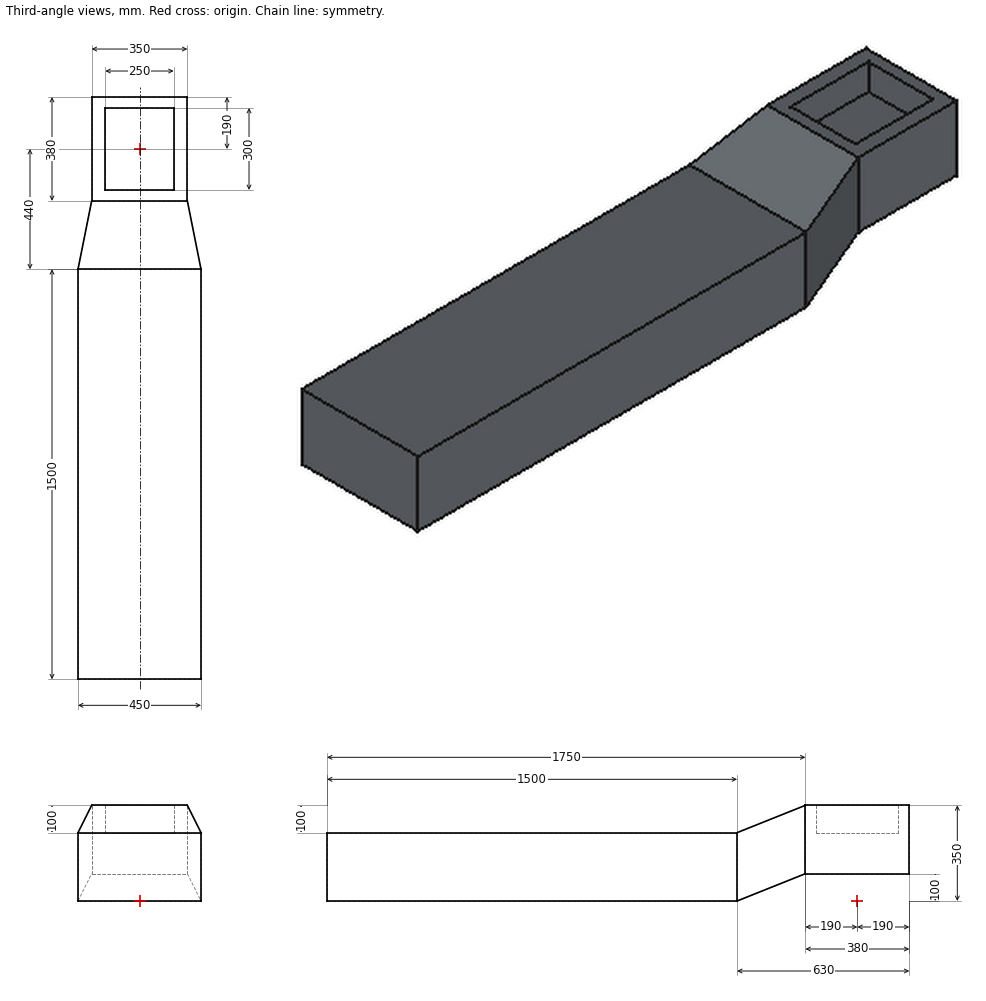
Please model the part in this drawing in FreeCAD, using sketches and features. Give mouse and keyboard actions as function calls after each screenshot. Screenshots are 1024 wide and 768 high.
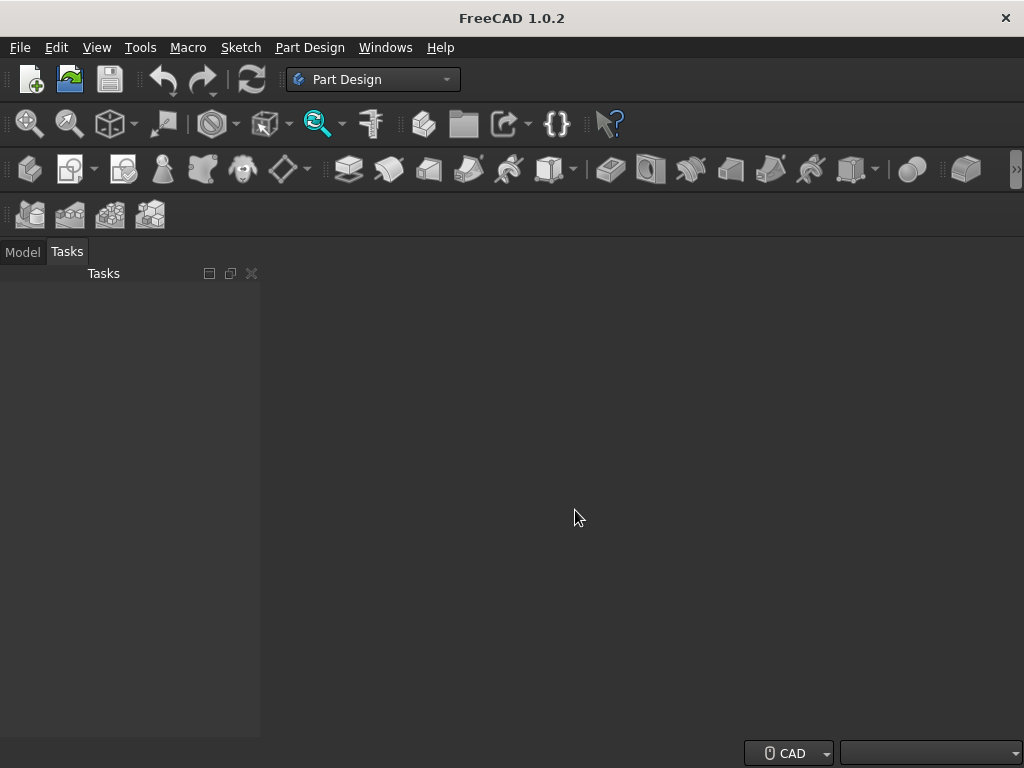
click(30, 80)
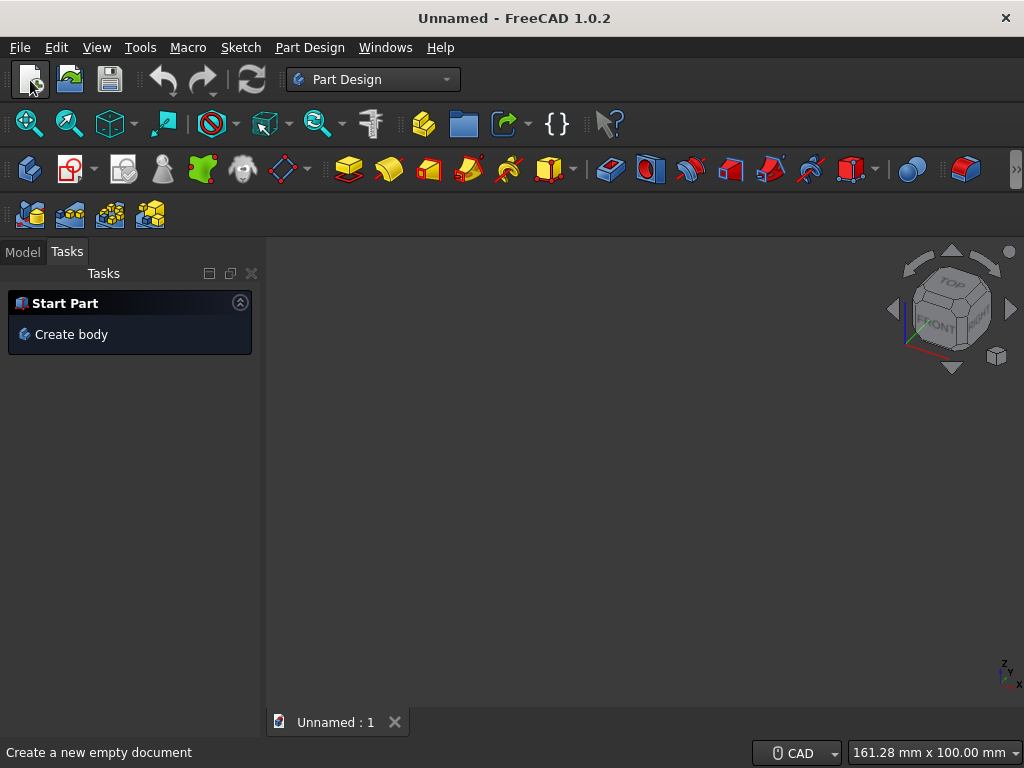
click(70, 170)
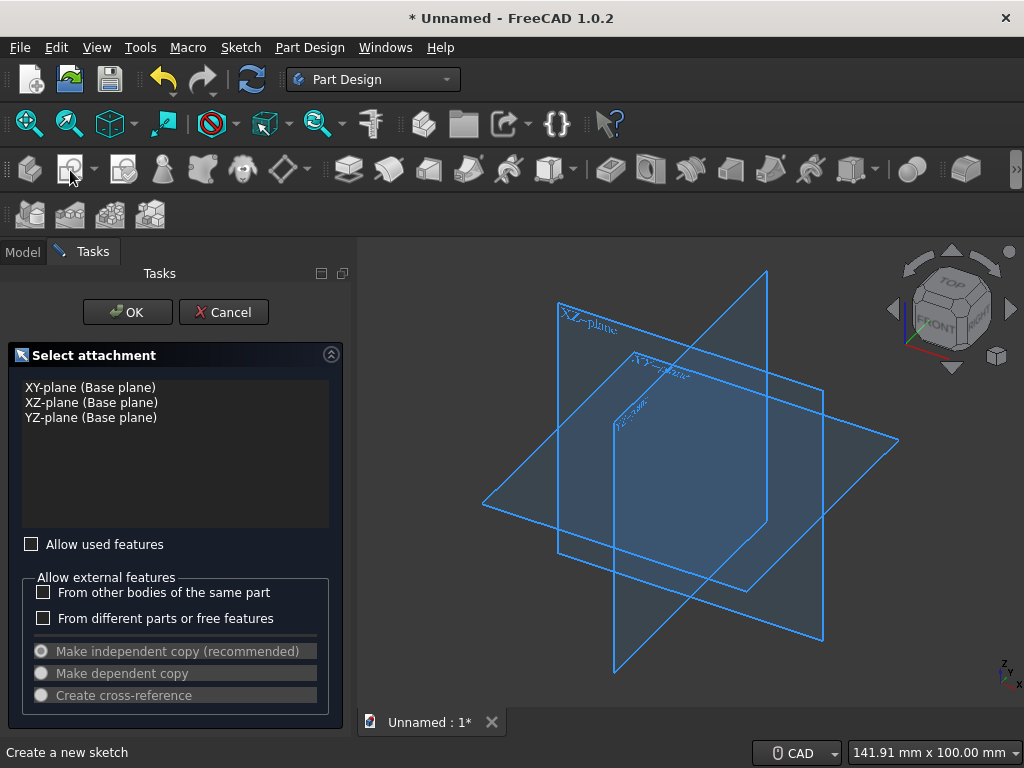
click(82, 388)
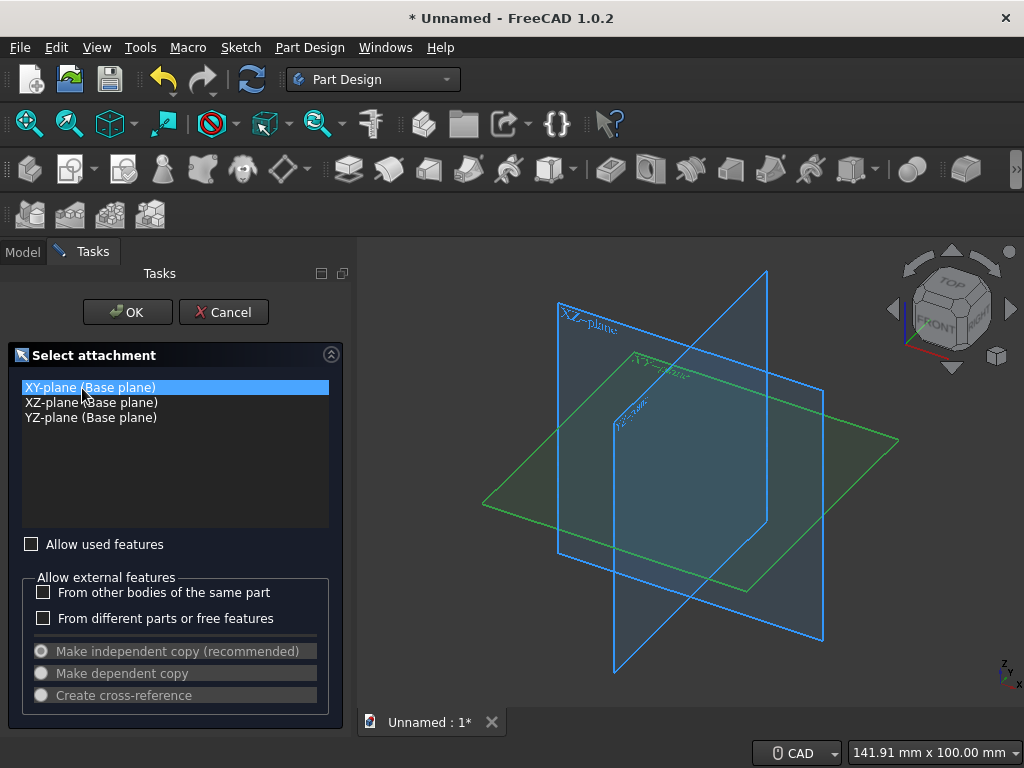
click(128, 312)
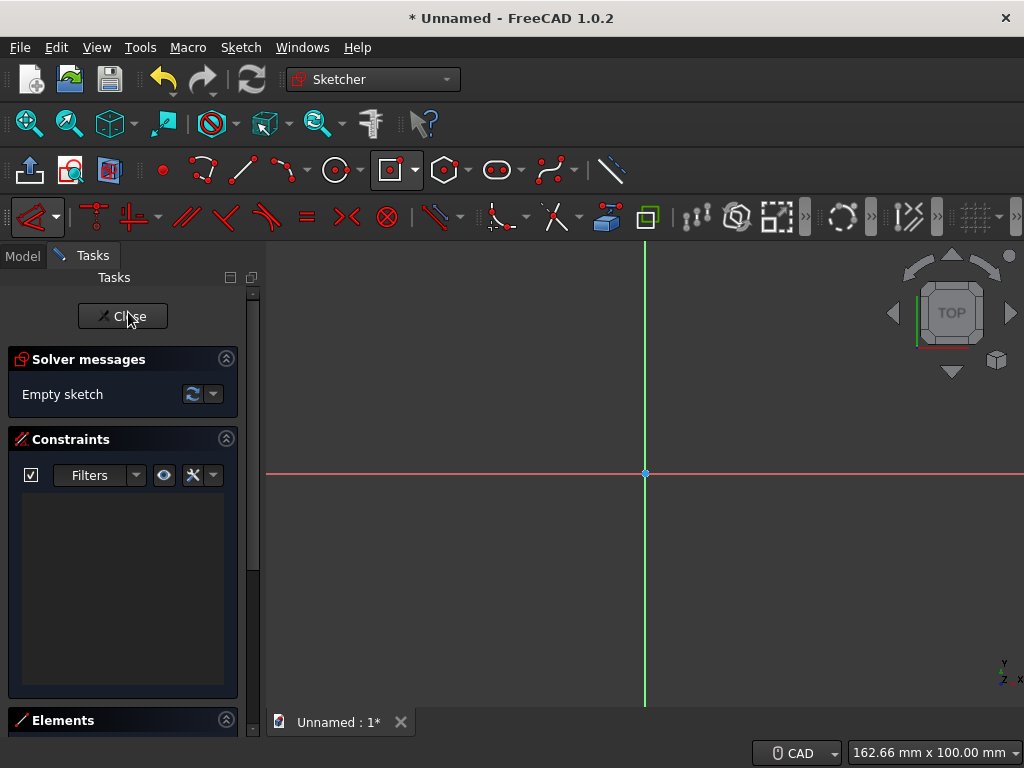
scroll(574, 333, down, 17)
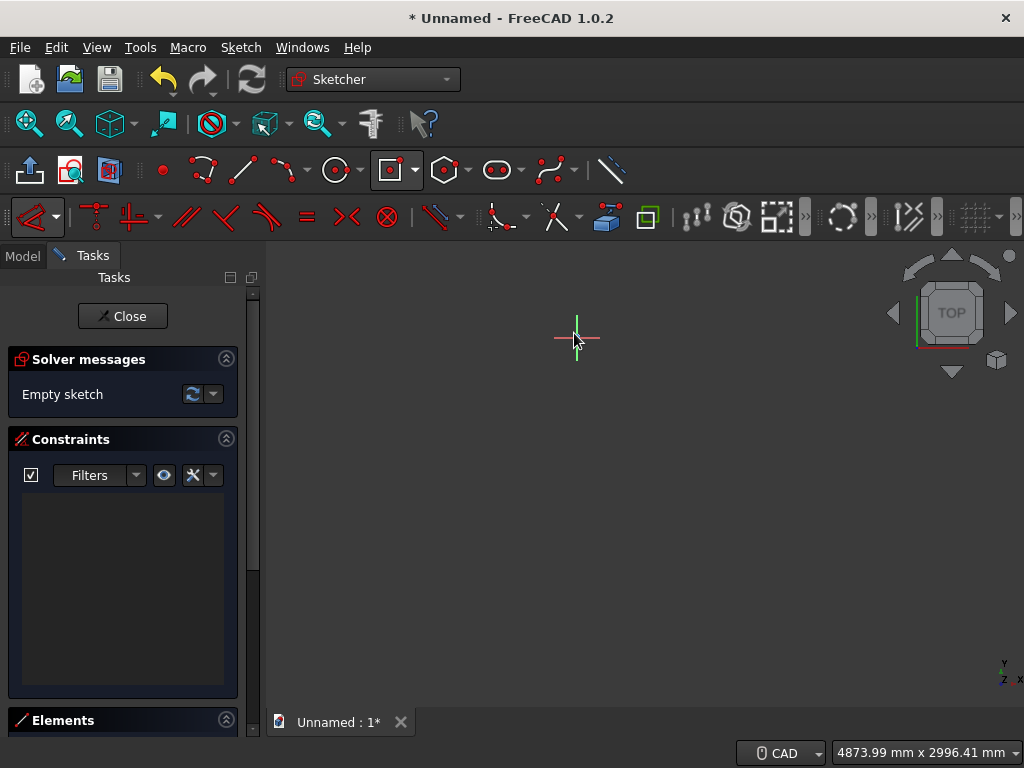
click(204, 170)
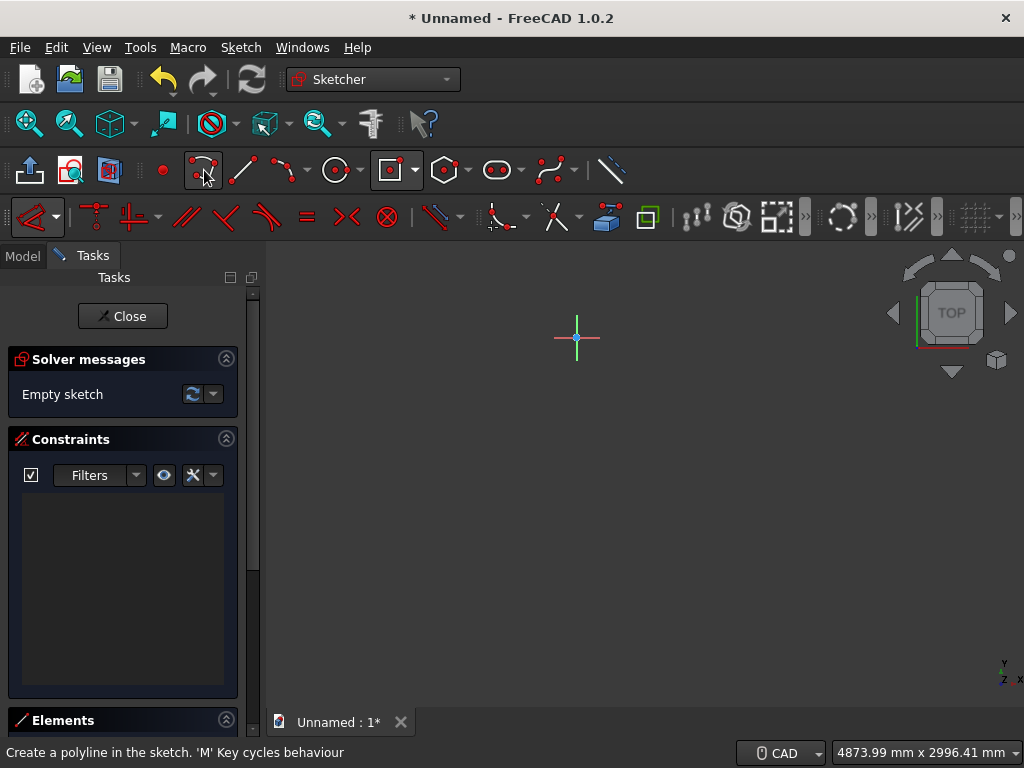
click(604, 308)
click(550, 308)
click(550, 367)
click(542, 406)
click(542, 640)
click(612, 640)
click(612, 406)
click(604, 367)
click(604, 309)
key(Escape)
key(Escape)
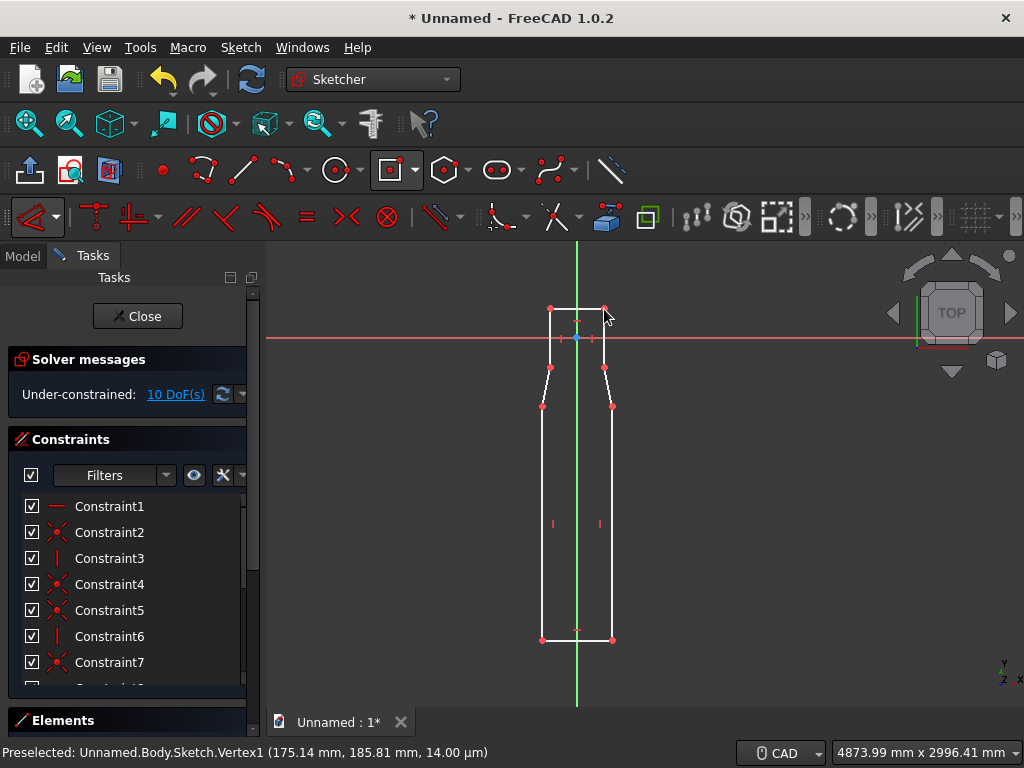
click(542, 407)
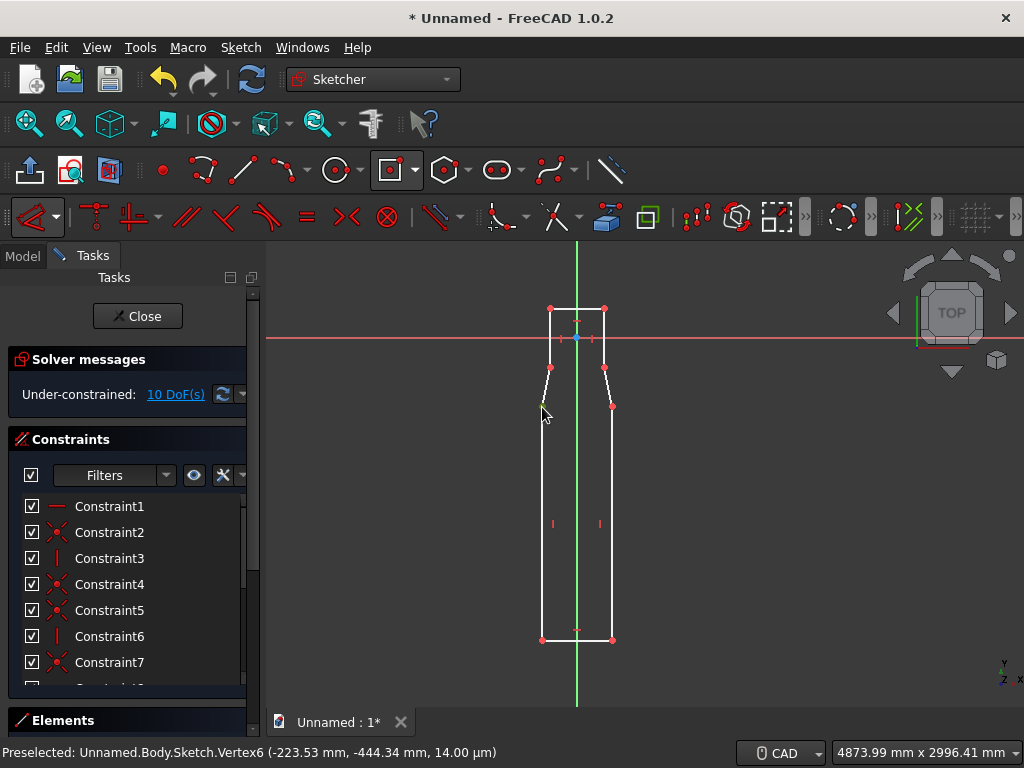
click(612, 407)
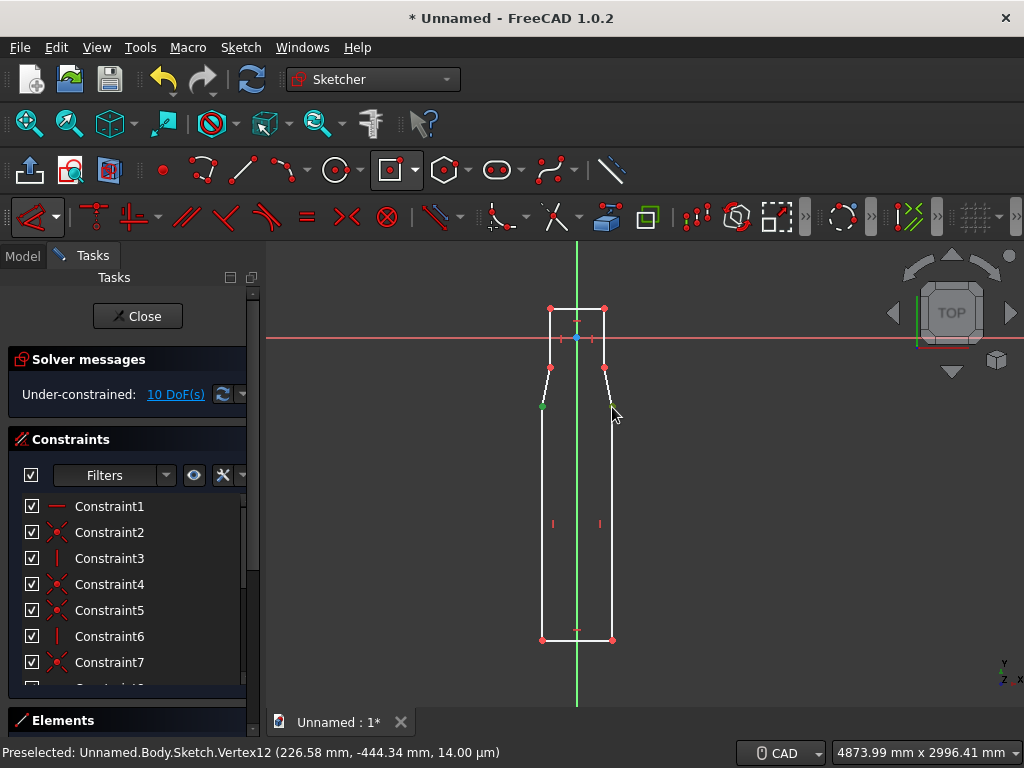
click(577, 591)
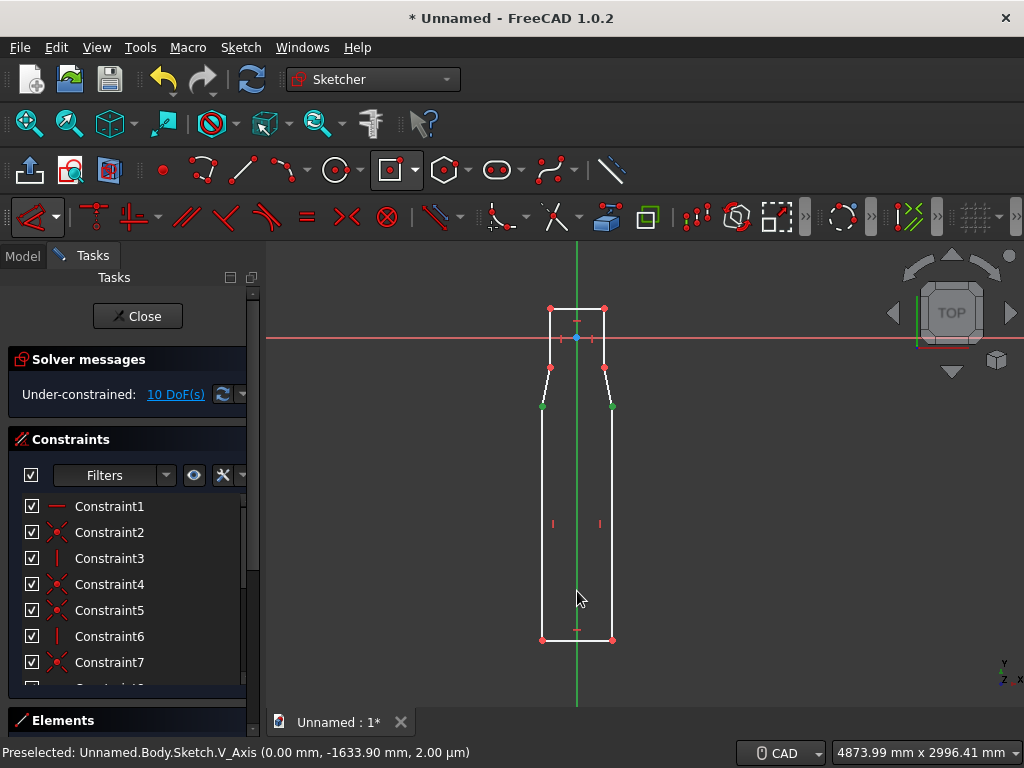
click(348, 218)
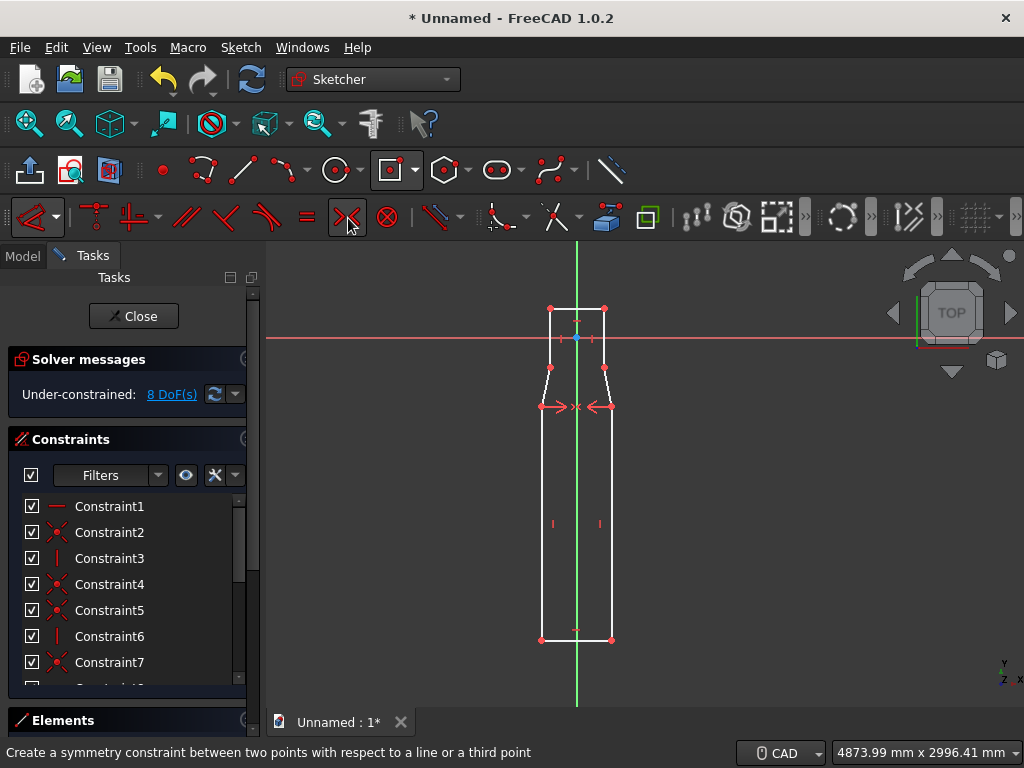
click(550, 368)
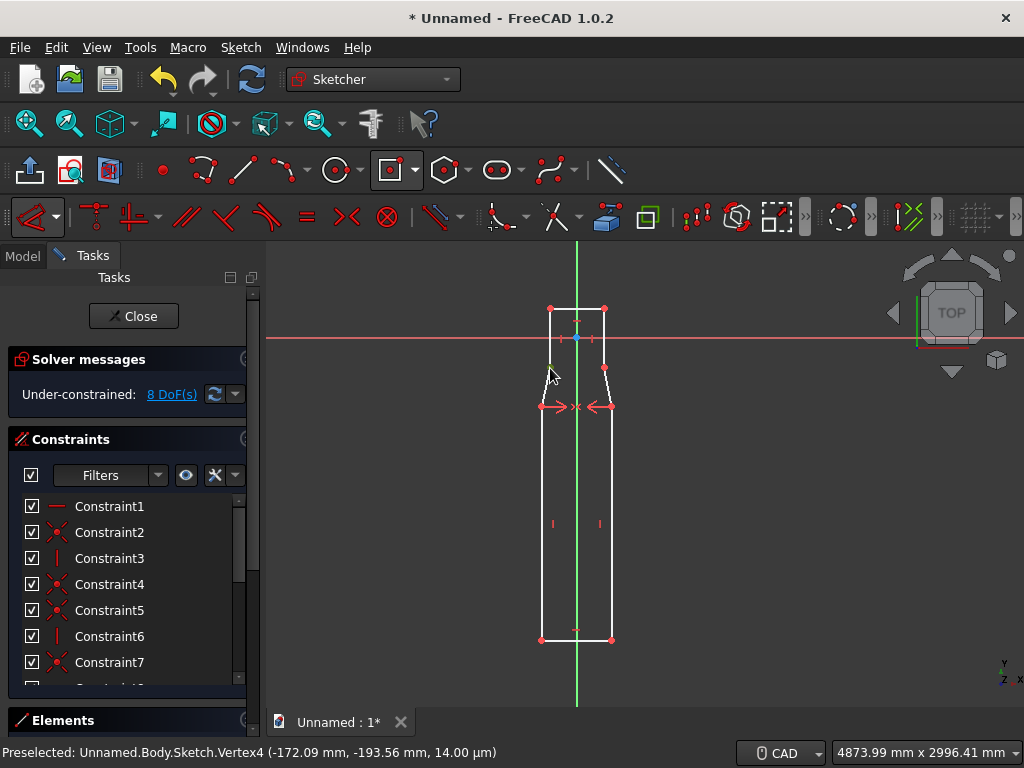
click(604, 368)